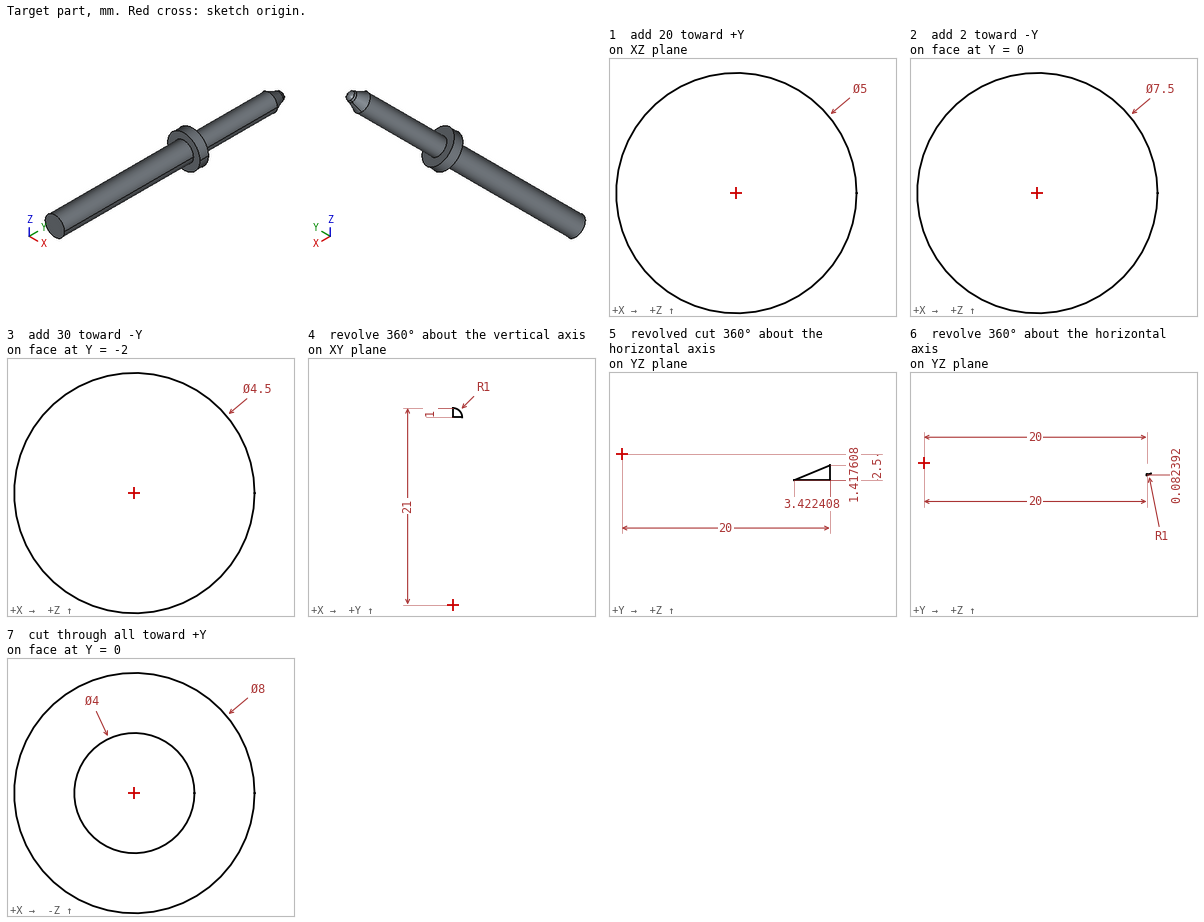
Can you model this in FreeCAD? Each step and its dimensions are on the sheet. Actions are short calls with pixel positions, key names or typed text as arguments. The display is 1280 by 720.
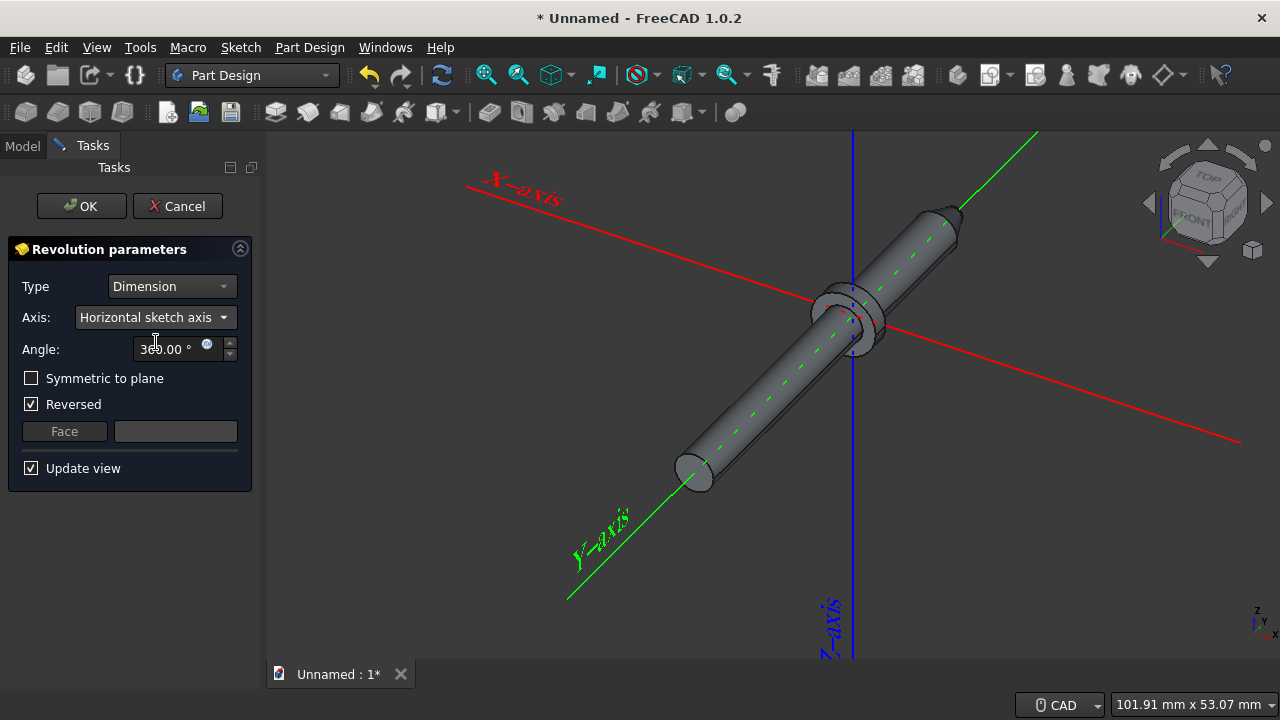
click(82, 206)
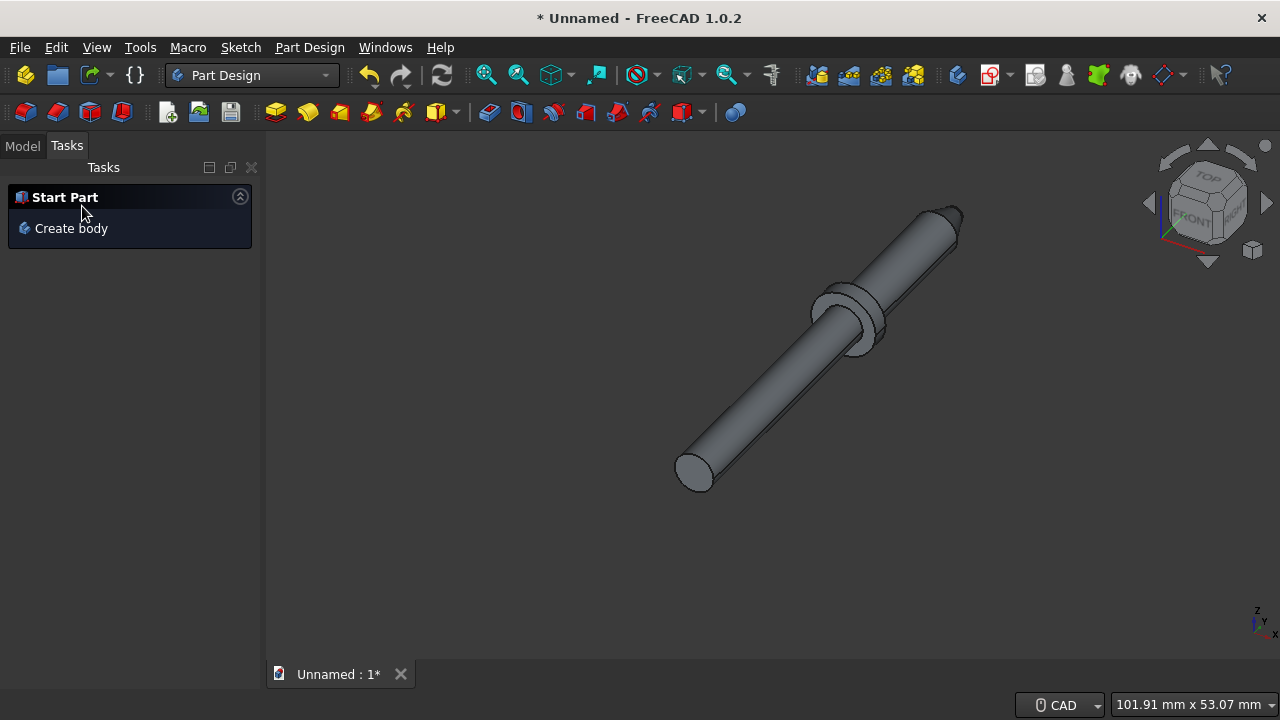
key(4)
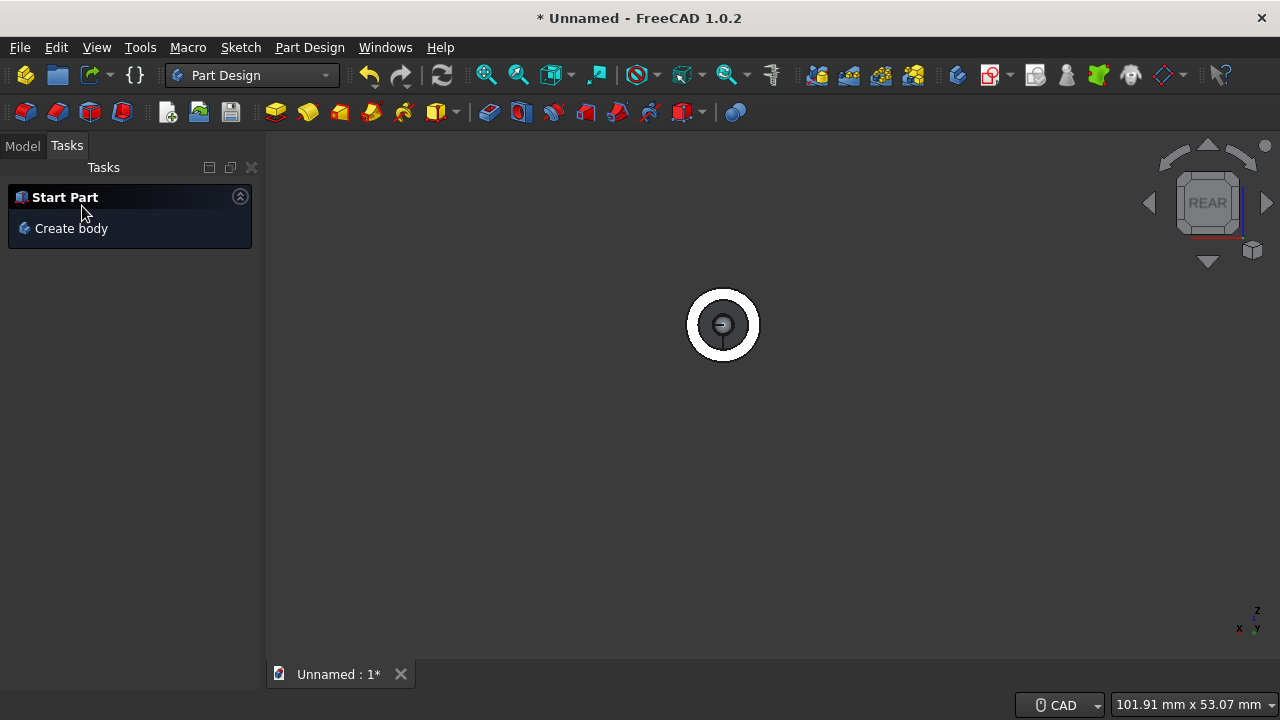
click(488, 76)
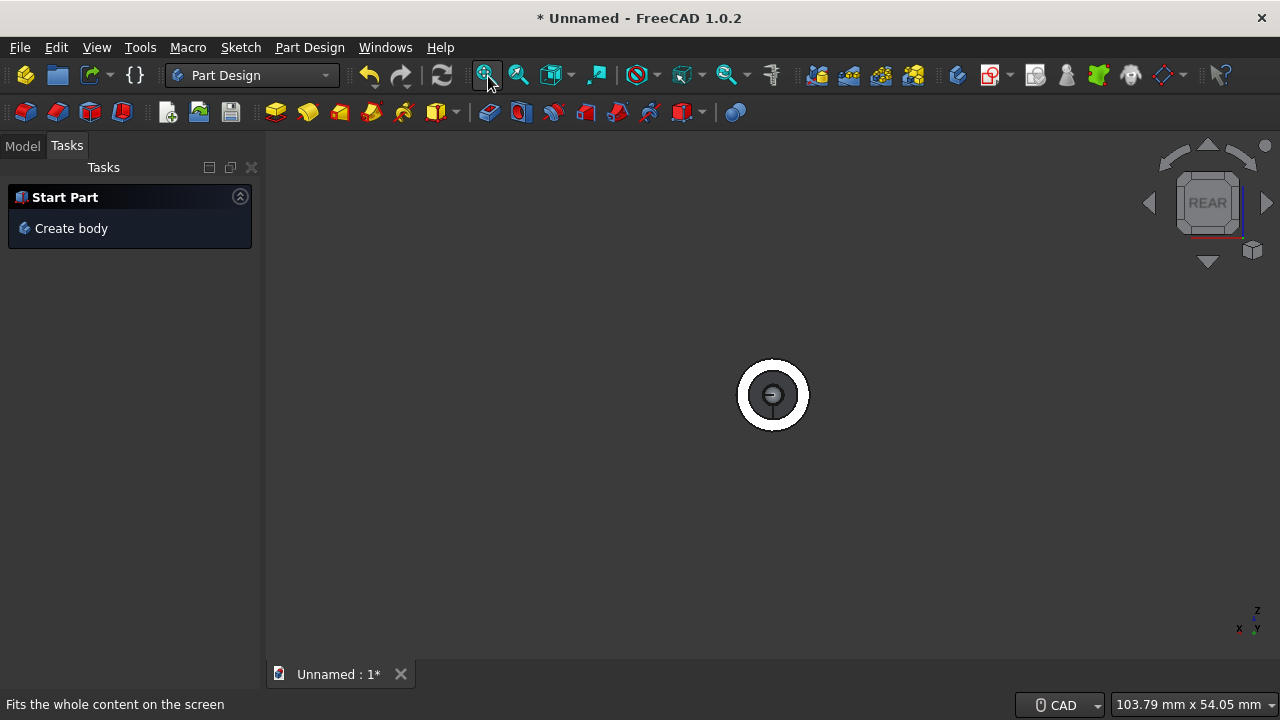
scroll(742, 394, up, 5)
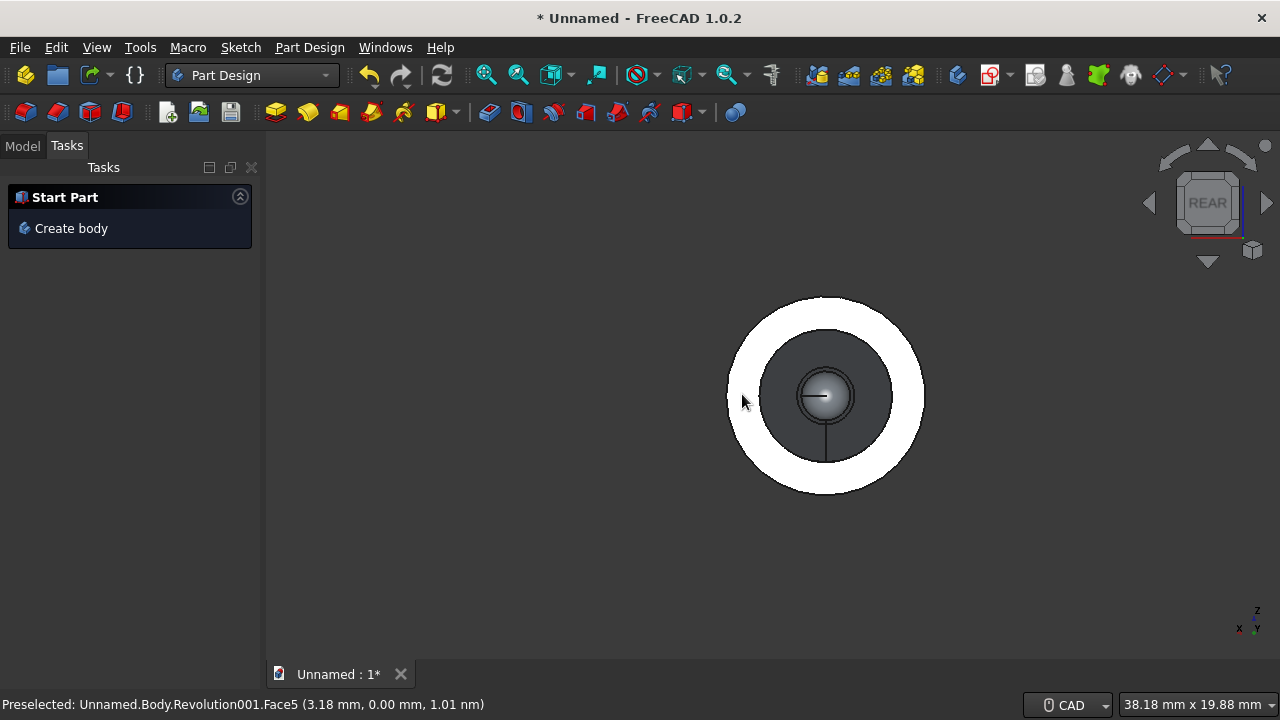
click(740, 395)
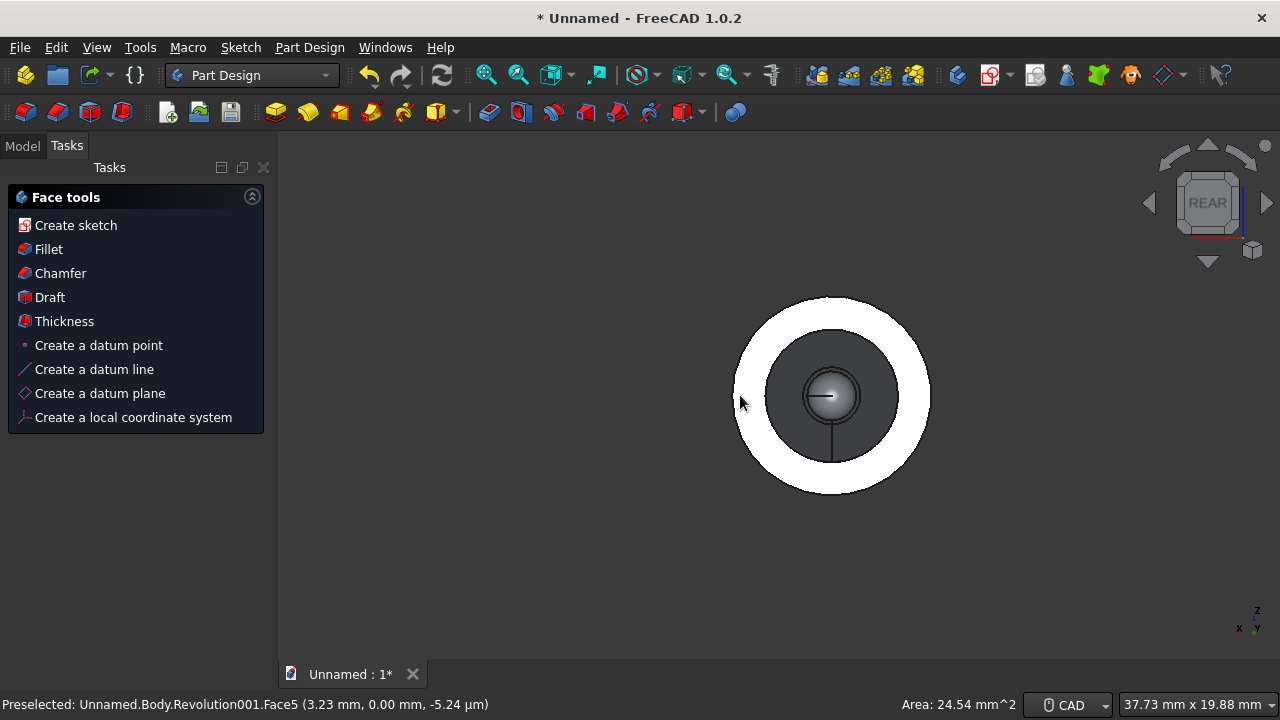
click(990, 76)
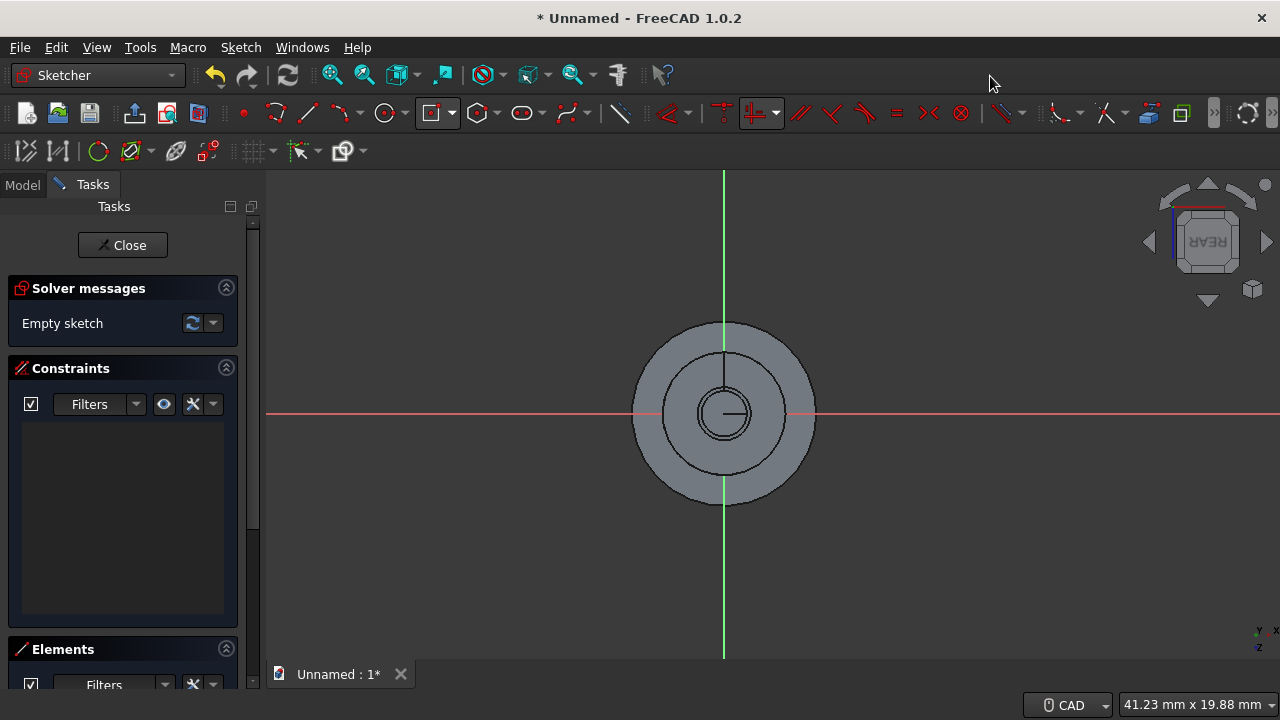
click(200, 114)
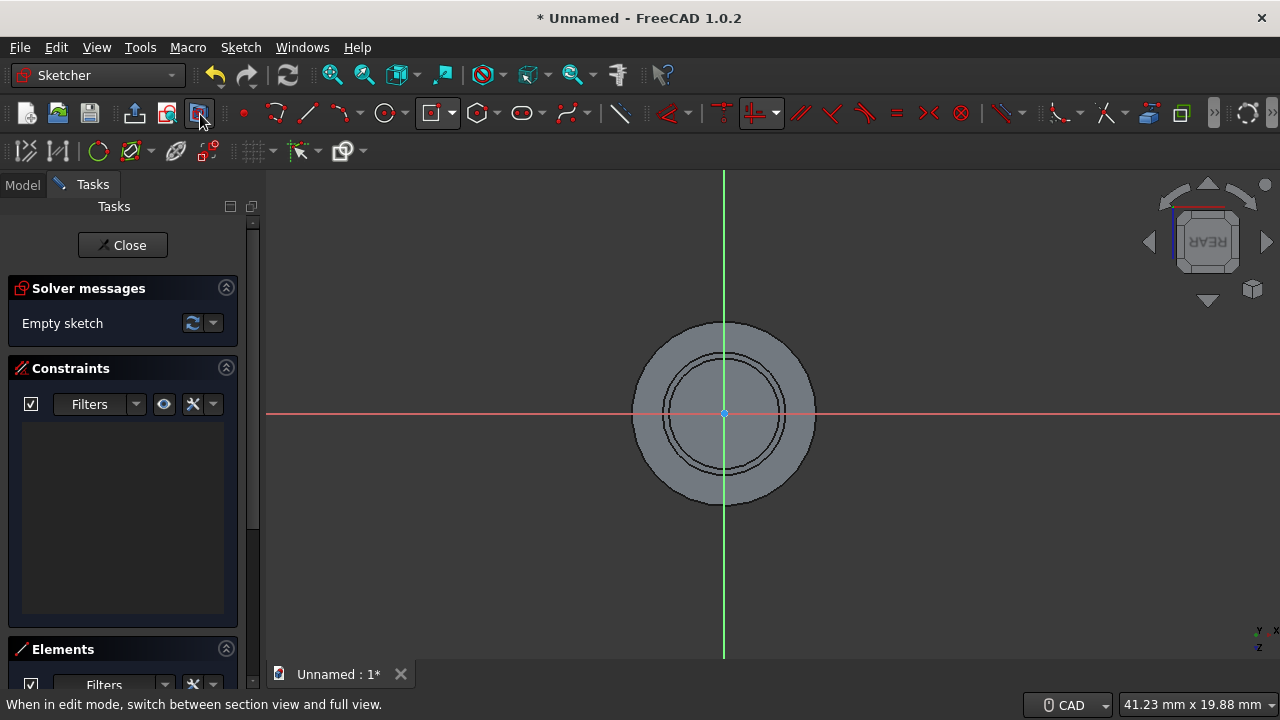
scroll(764, 412, up, 2)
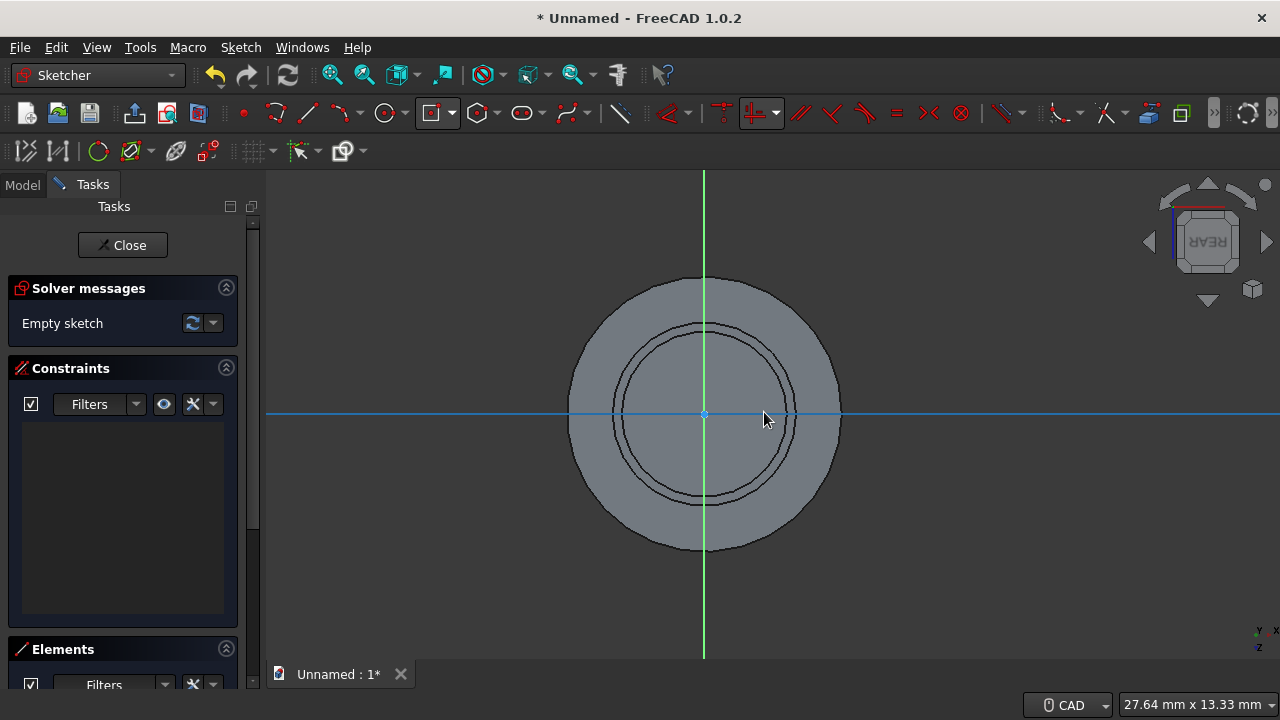
click(386, 114)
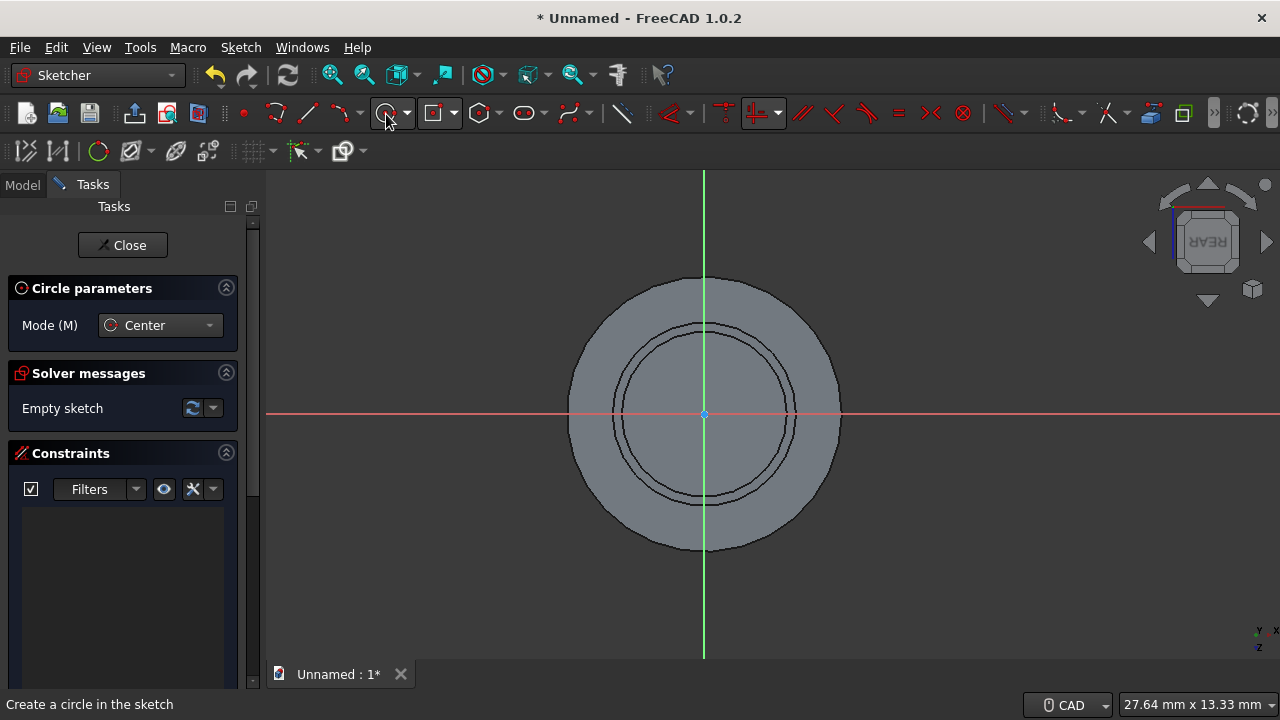
click(704, 414)
click(808, 311)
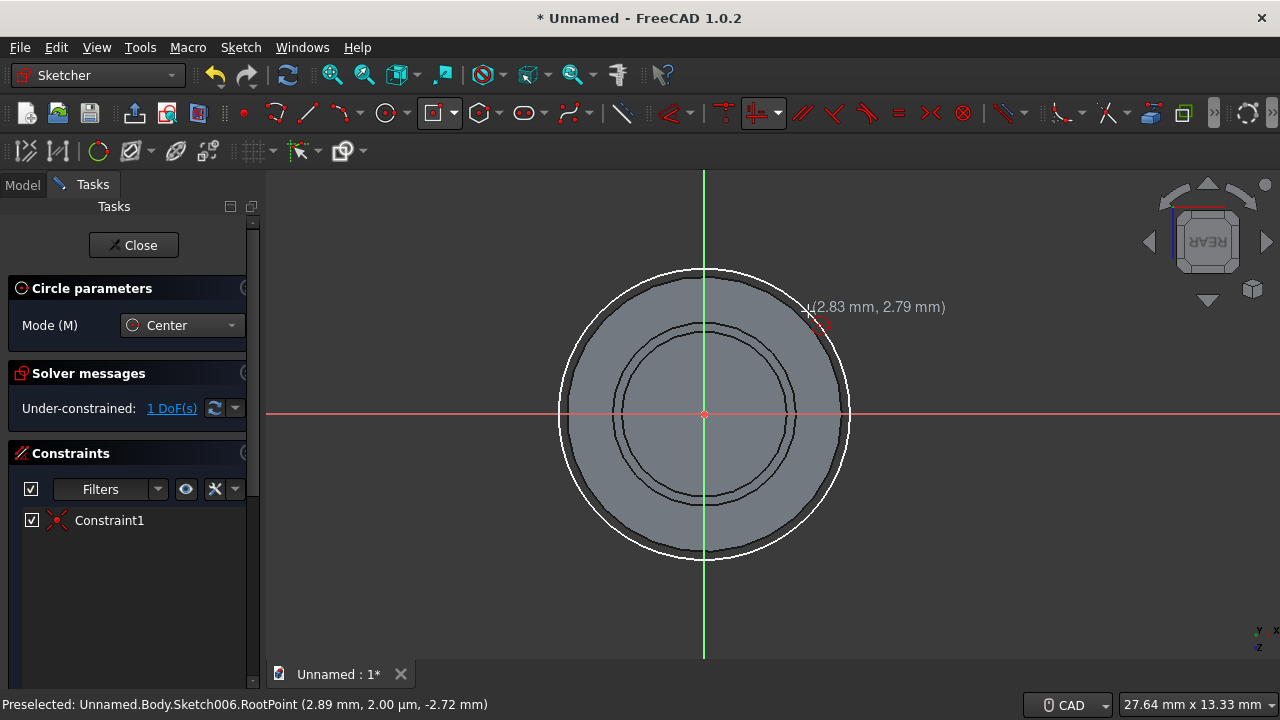
click(704, 414)
click(756, 362)
key(Escape)